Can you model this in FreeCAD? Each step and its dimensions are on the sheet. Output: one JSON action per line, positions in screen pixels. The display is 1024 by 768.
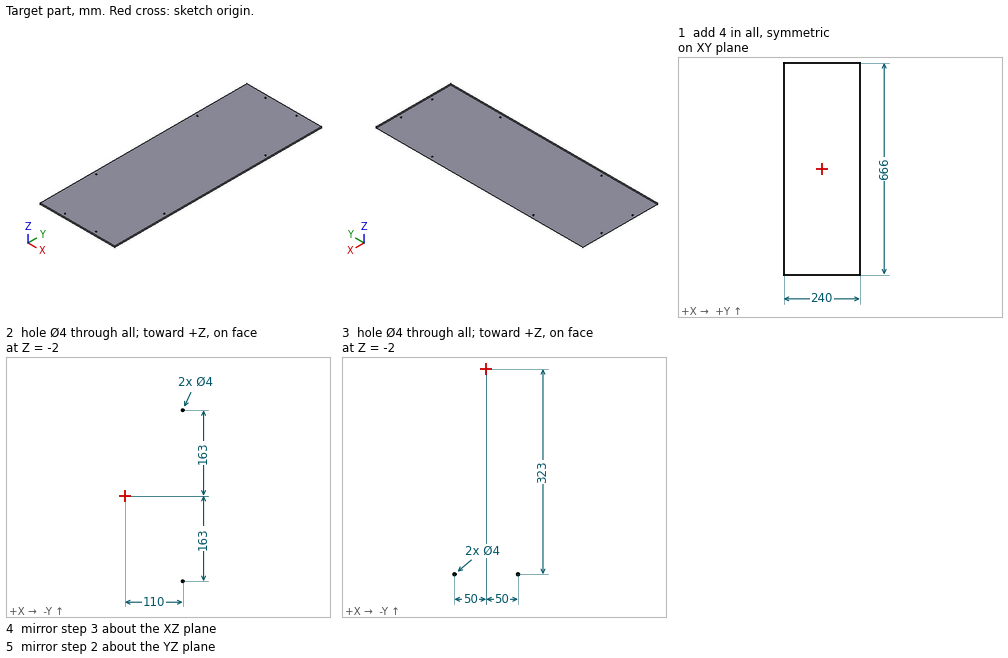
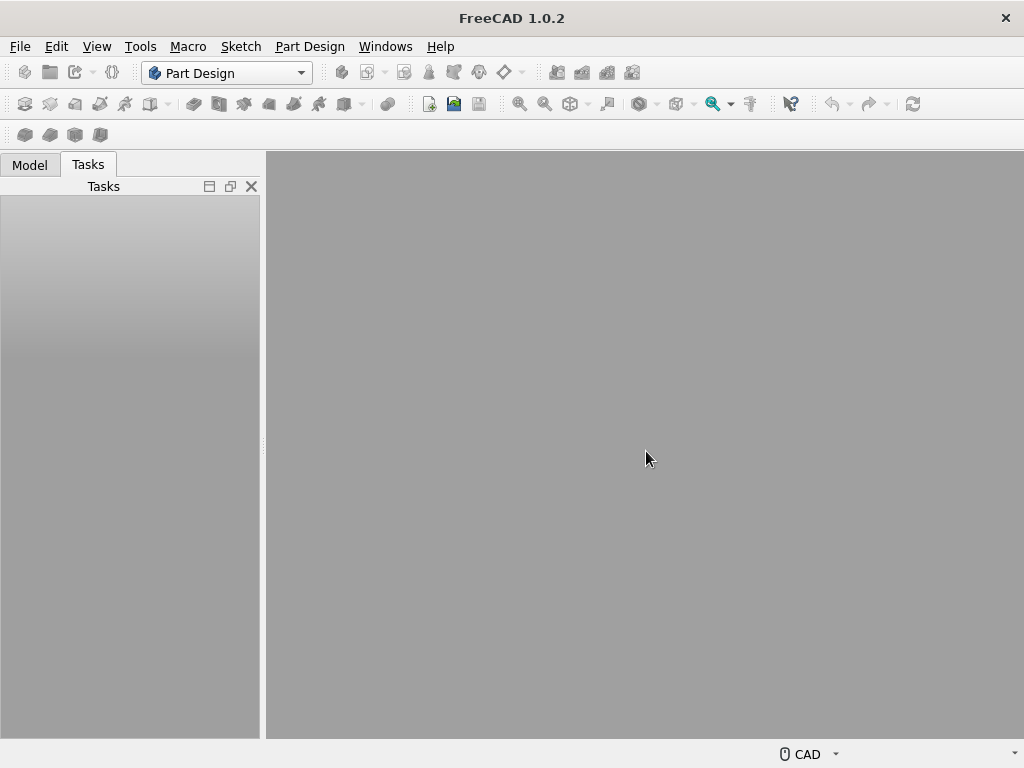
{"action": "left_click", "coordinate": [429, 104]}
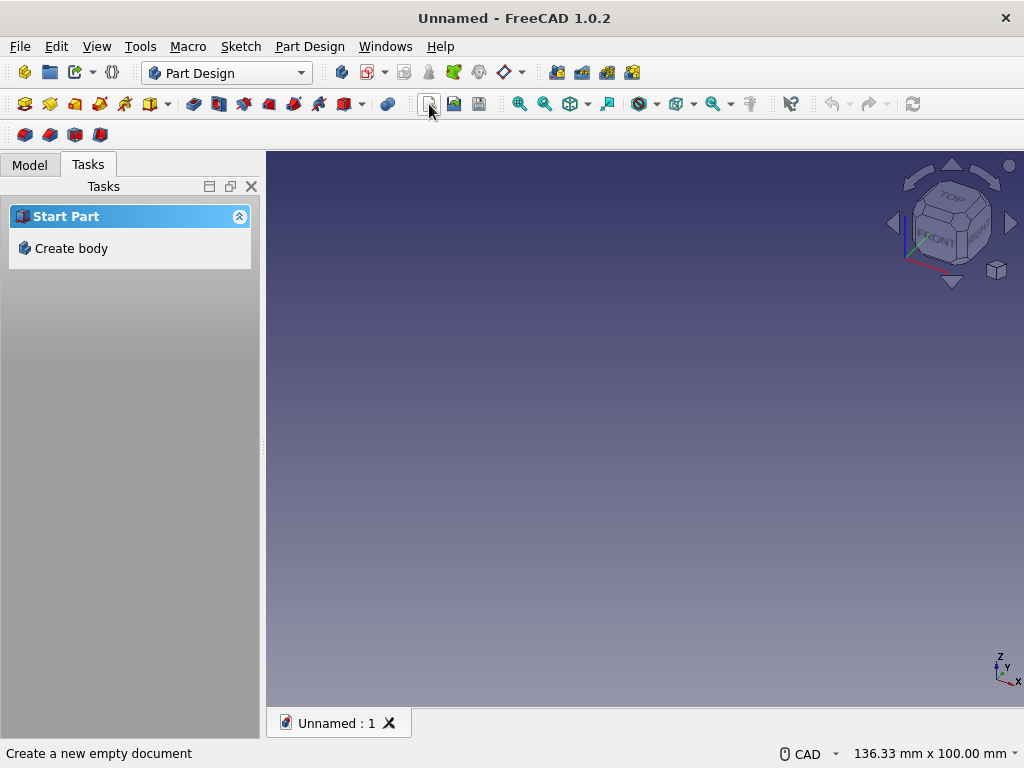
{"action": "left_click", "coordinate": [366, 72]}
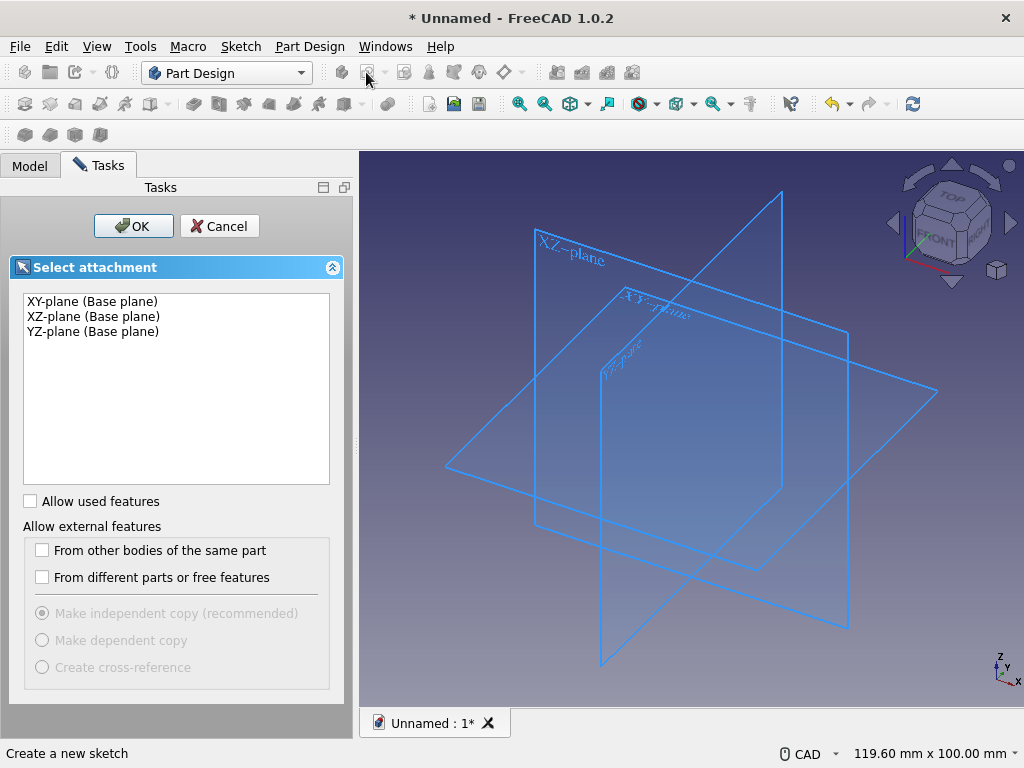
{"action": "left_click", "coordinate": [84, 302]}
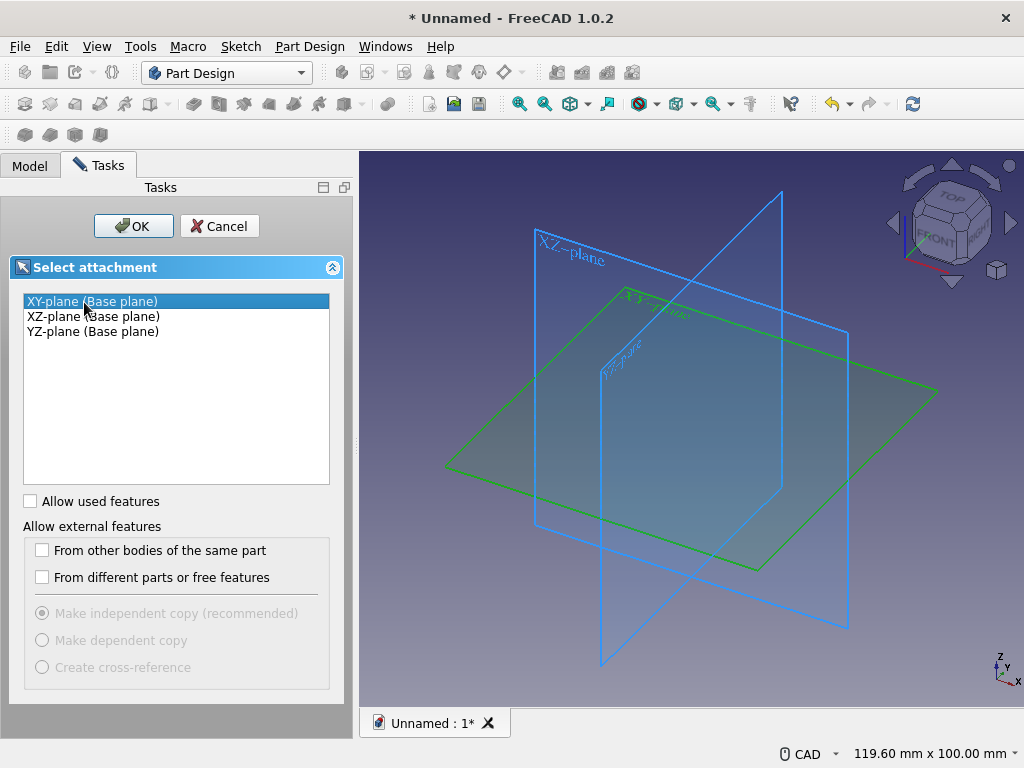
{"action": "left_click", "coordinate": [134, 226]}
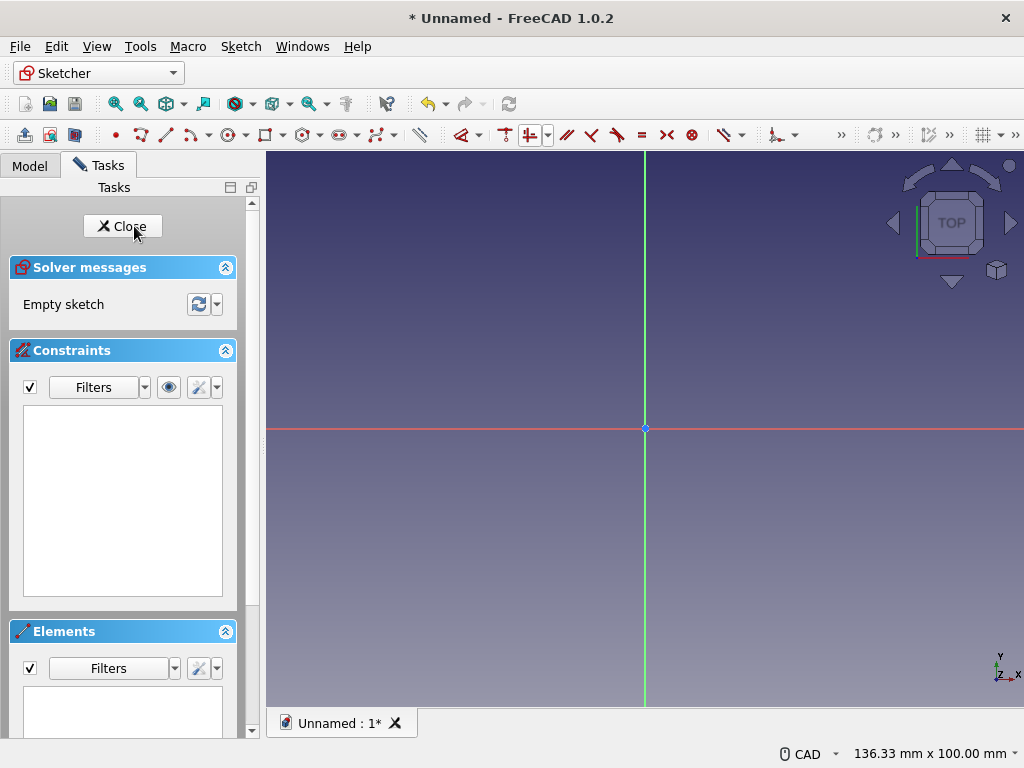
{"action": "scroll", "coordinate": [570, 429], "scroll_direction": "down", "scroll_amount": 12}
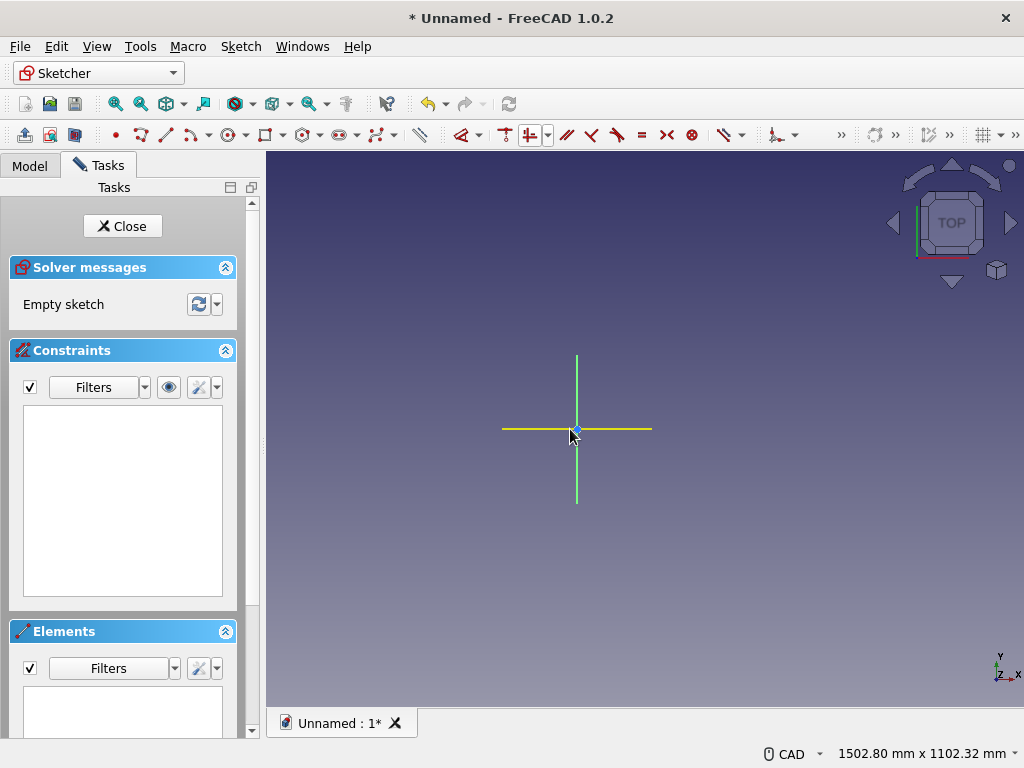
{"action": "left_click", "coordinate": [282, 136]}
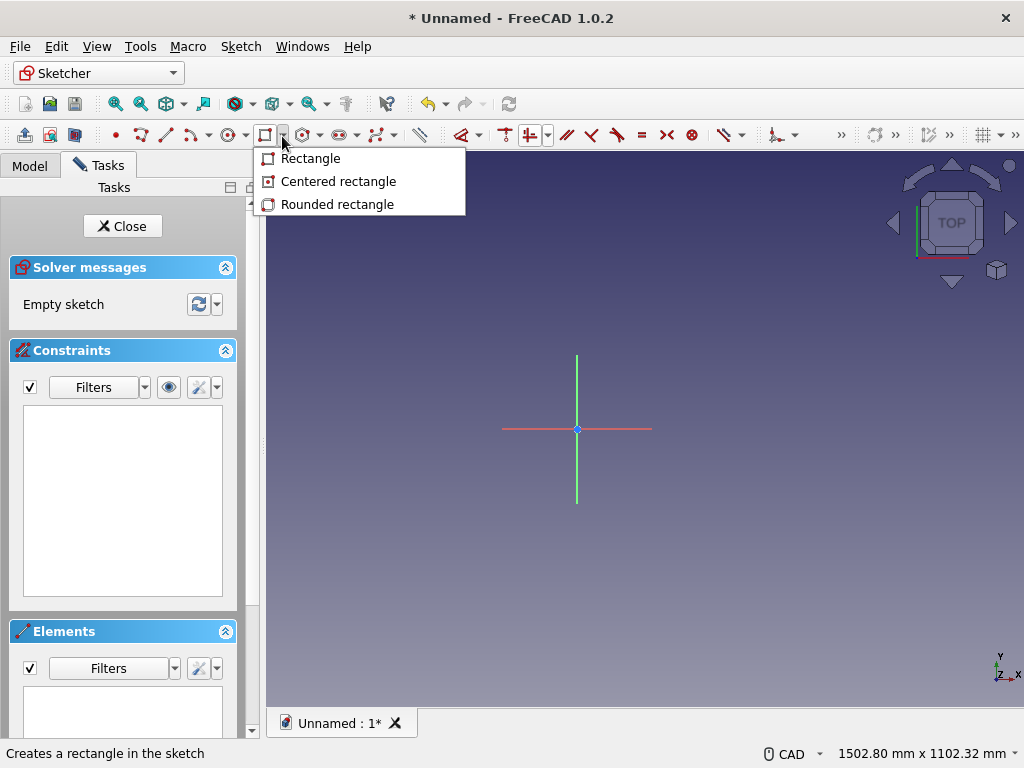
{"action": "left_click", "coordinate": [360, 182]}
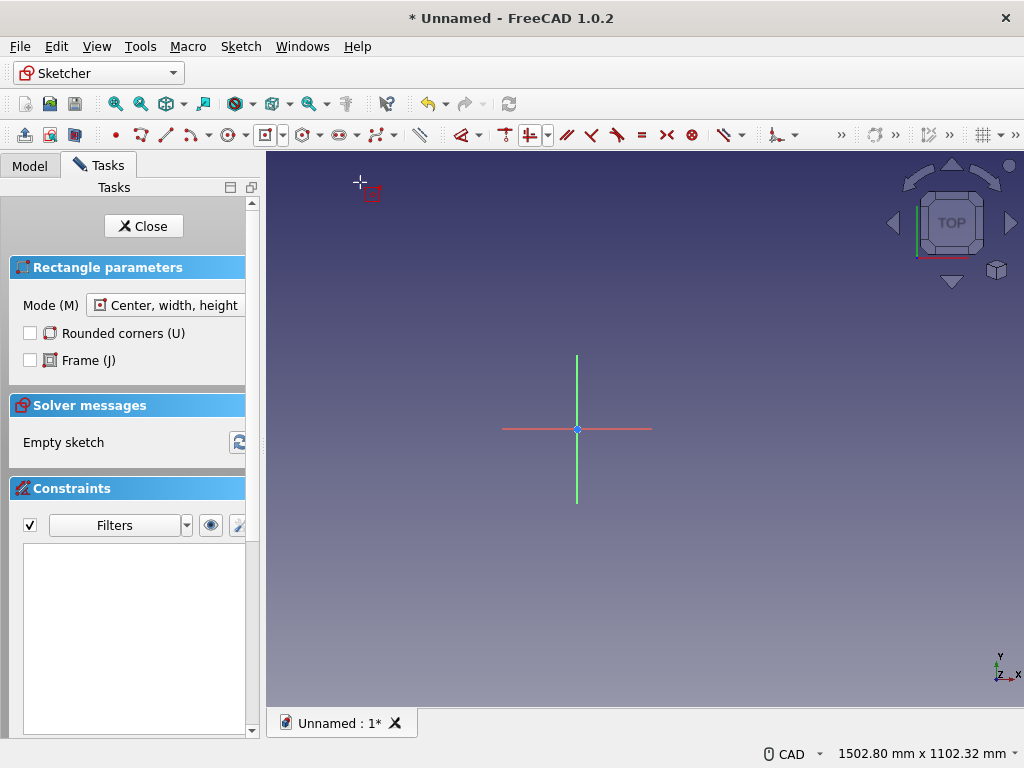
{"action": "left_click", "coordinate": [577, 429]}
{"action": "left_click", "coordinate": [638, 261]}
{"action": "key", "text": "Escape"}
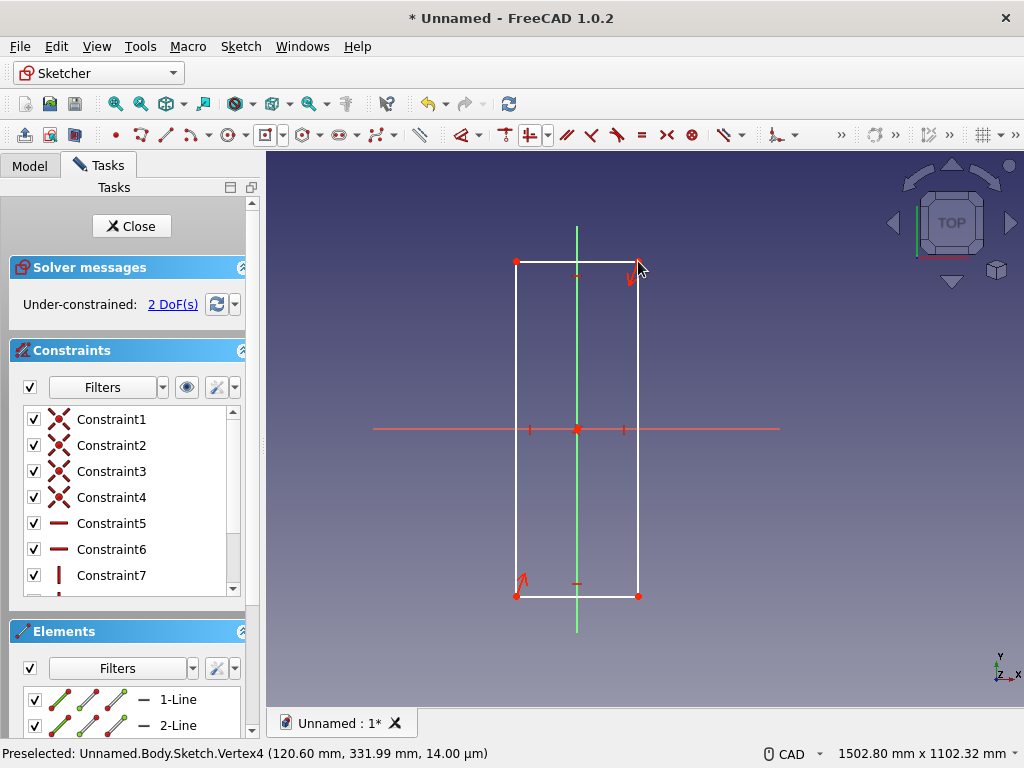
{"action": "left_click", "coordinate": [460, 136]}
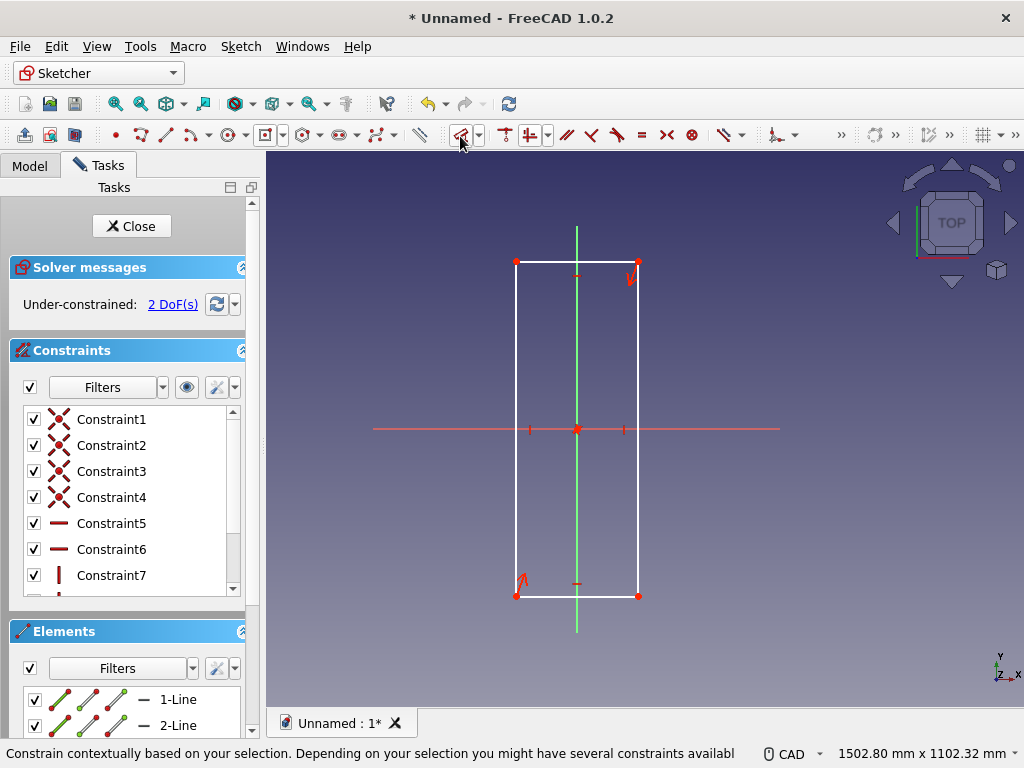
{"action": "left_click", "coordinate": [553, 597]}
{"action": "left_click", "coordinate": [549, 631]}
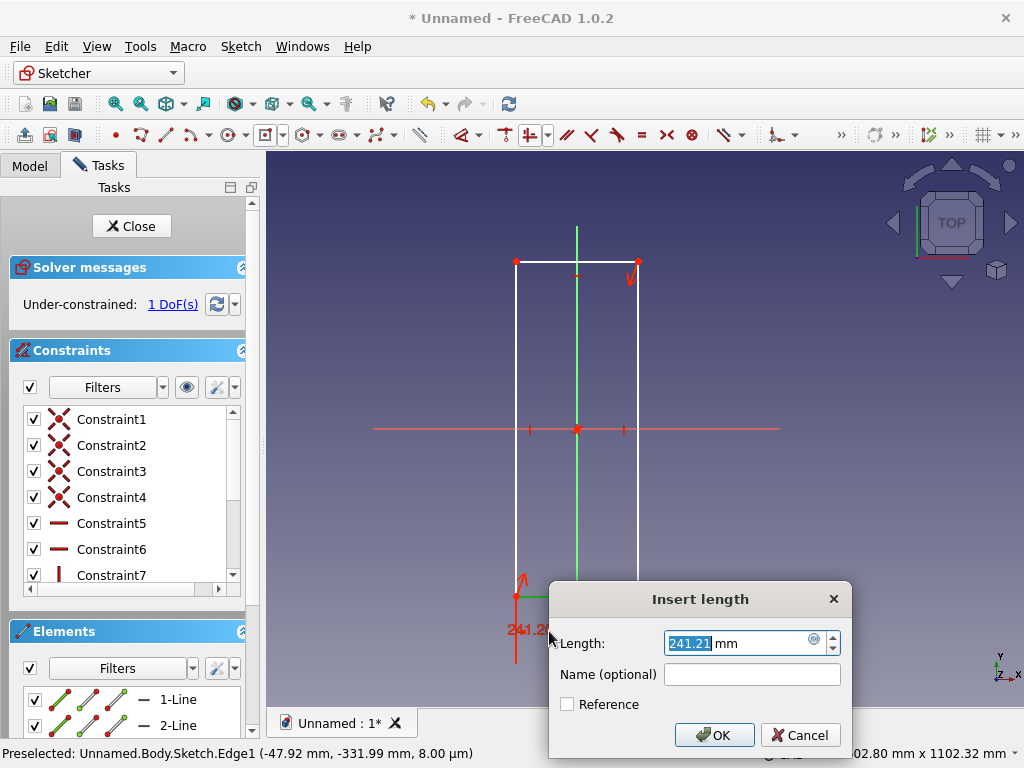
{"action": "type", "text": "240"}
{"action": "key", "text": "Return"}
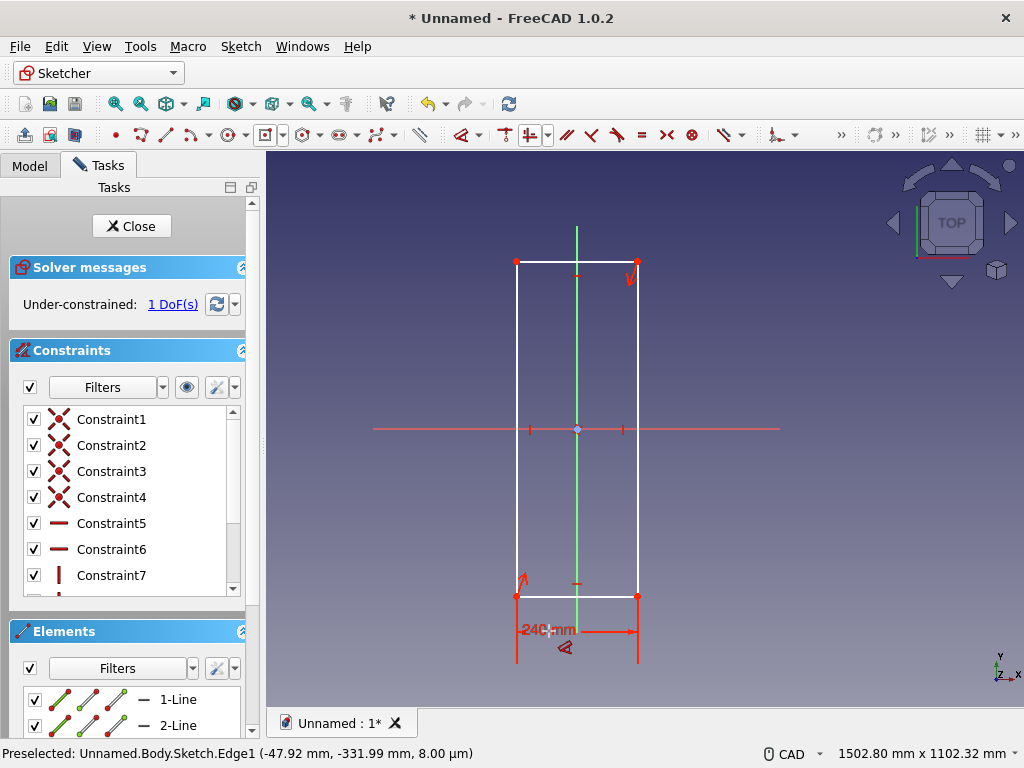
{"action": "left_click", "coordinate": [638, 496]}
{"action": "left_click", "coordinate": [672, 352]}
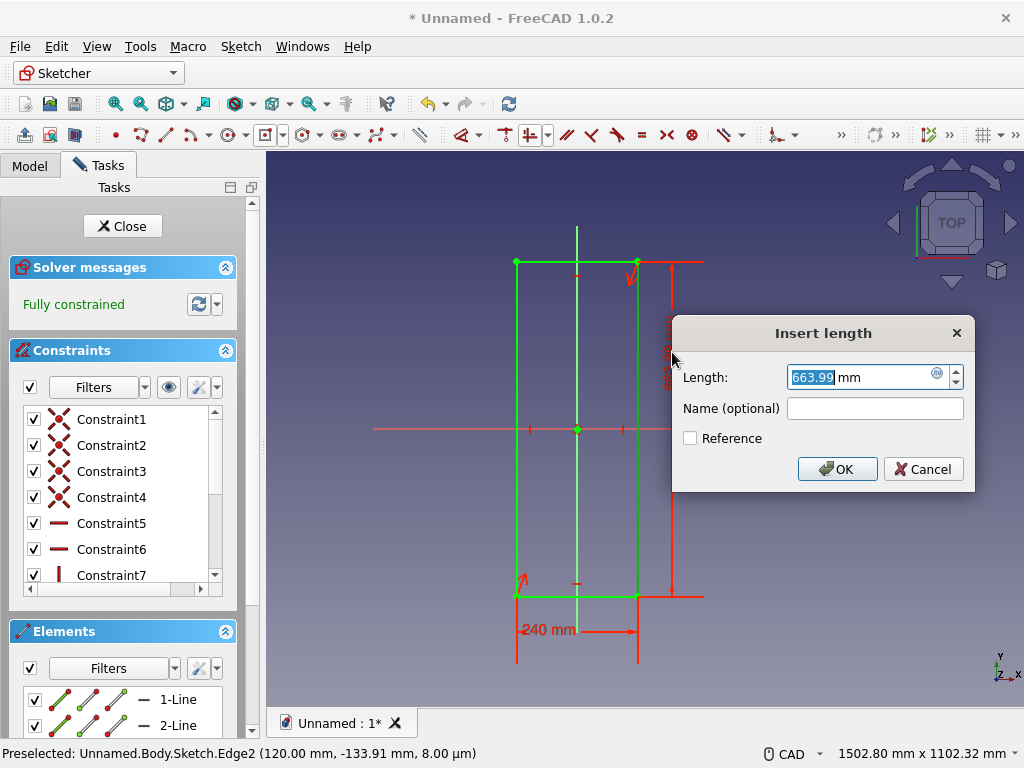
{"action": "type", "text": "666"}
{"action": "key", "text": "Return"}
{"action": "key", "text": "Escape"}